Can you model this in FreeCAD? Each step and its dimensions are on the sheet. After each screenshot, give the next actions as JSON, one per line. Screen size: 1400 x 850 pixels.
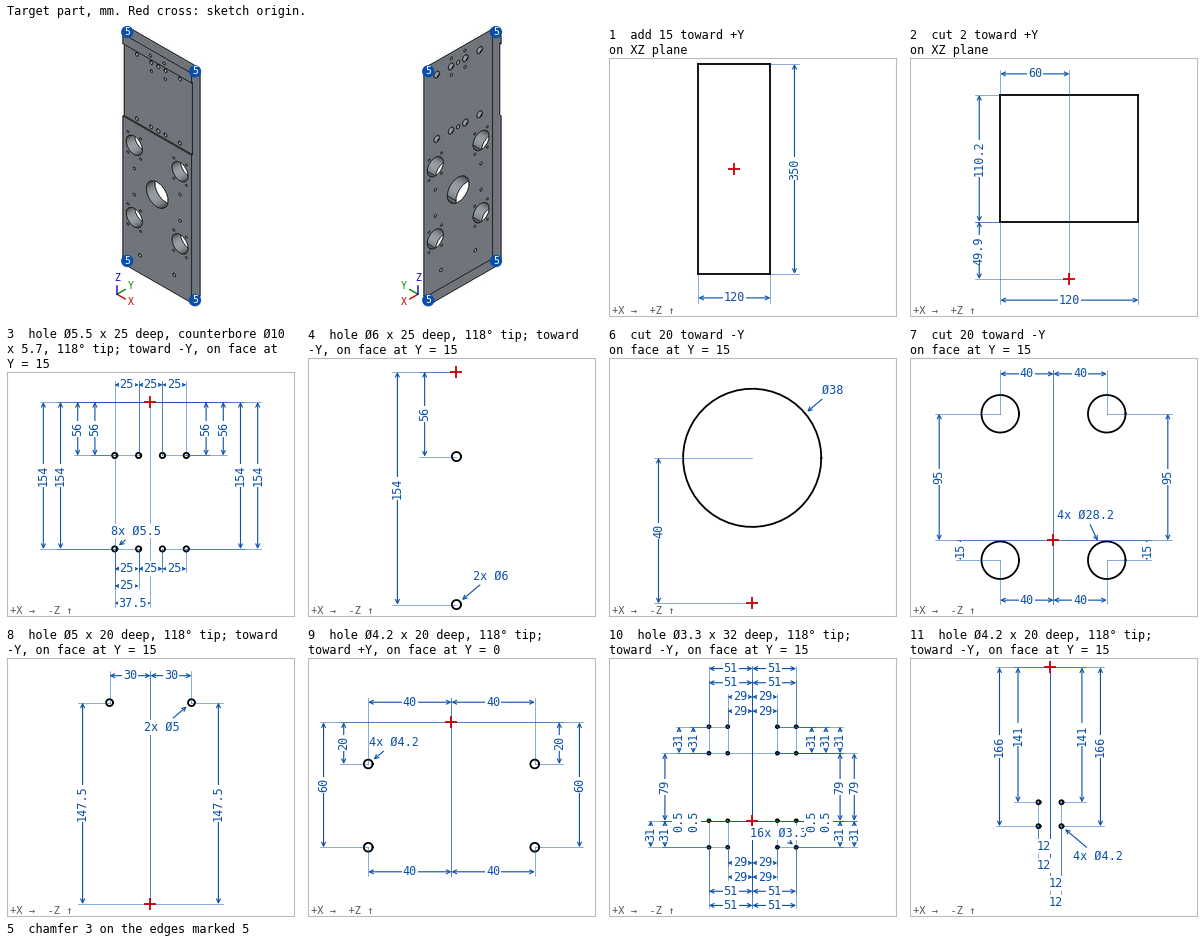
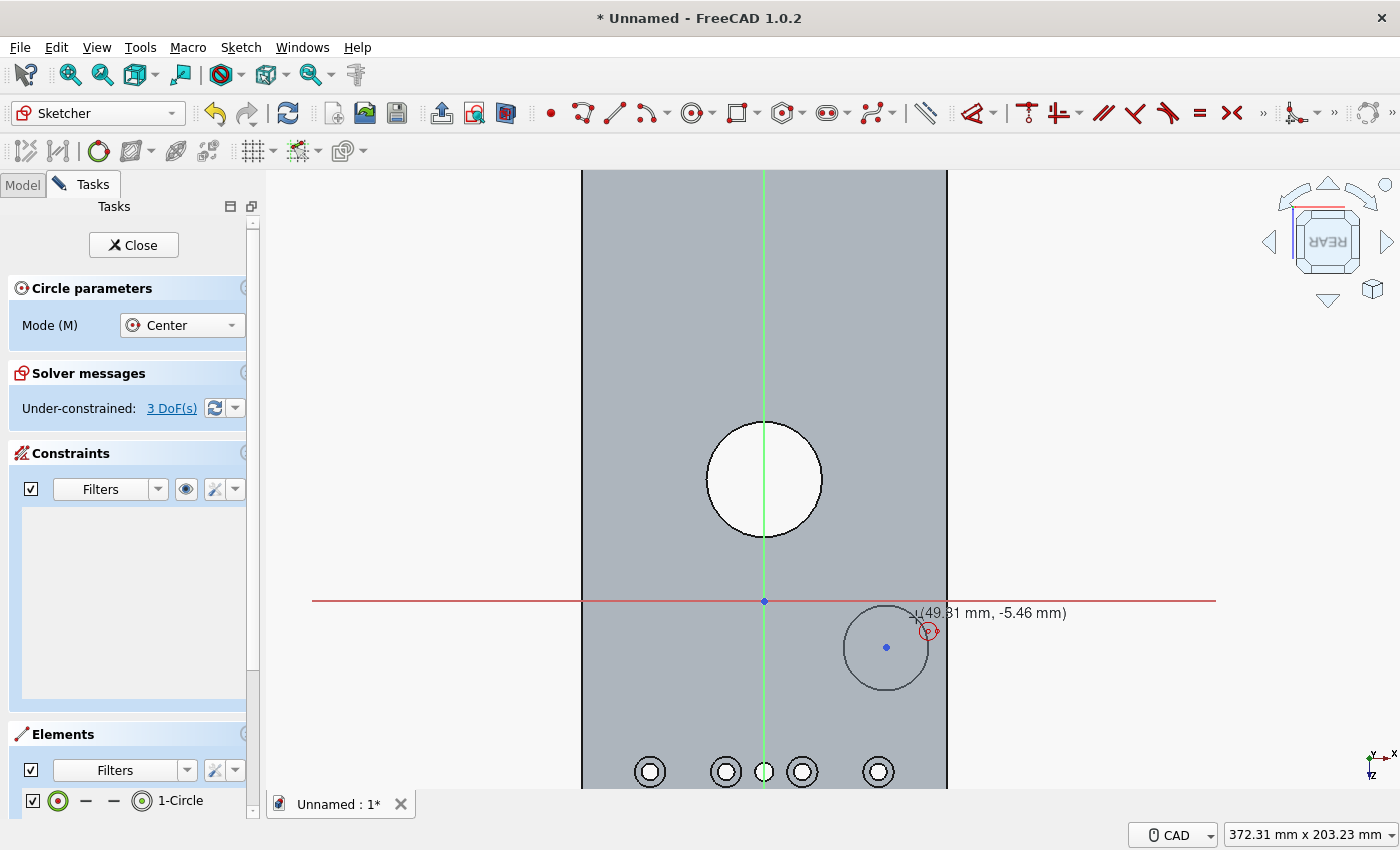
{"action": "left_click", "coordinate": [886, 312]}
{"action": "left_click", "coordinate": [916, 282]}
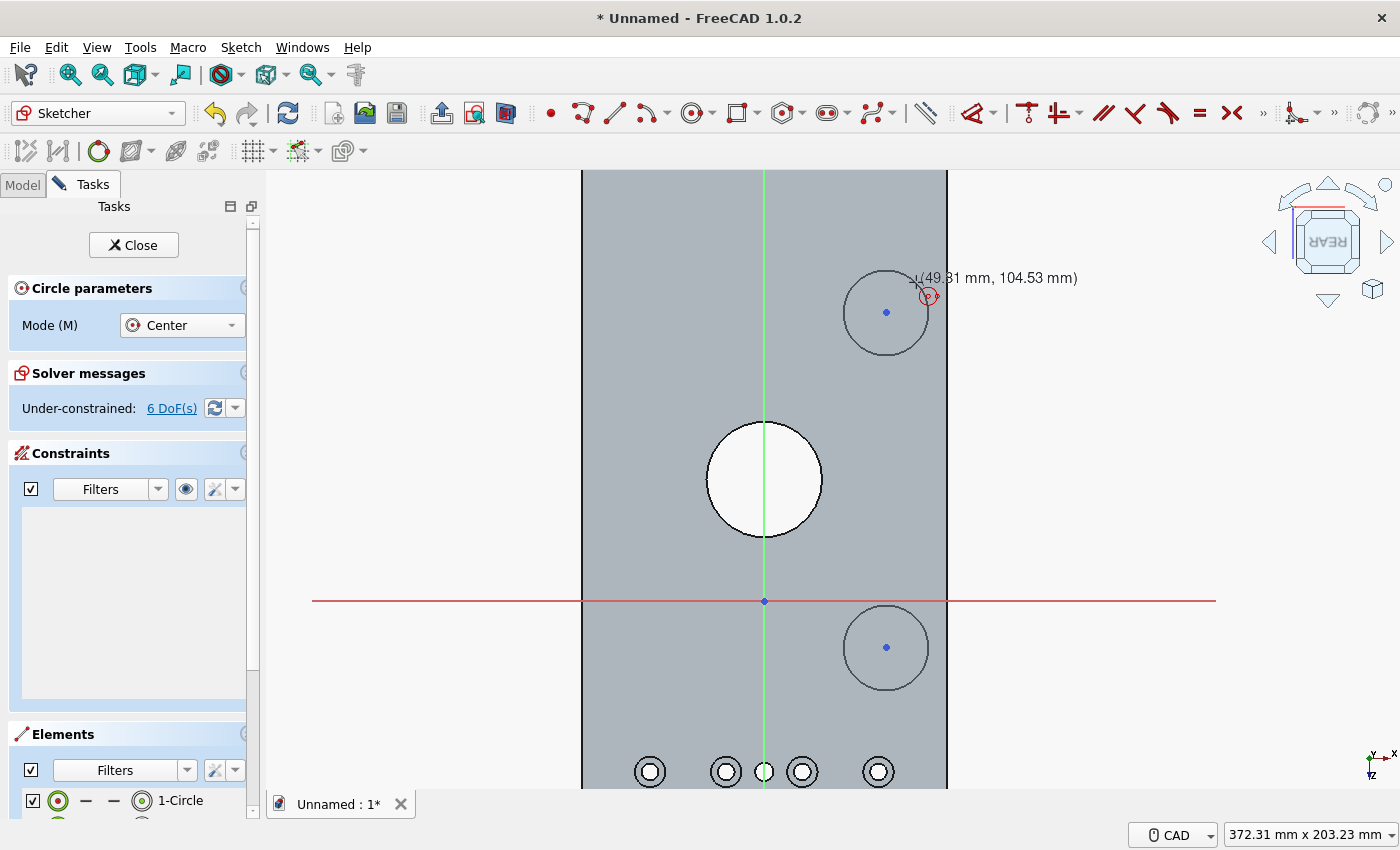
{"action": "left_click", "coordinate": [642, 647]}
{"action": "left_click", "coordinate": [673, 617]}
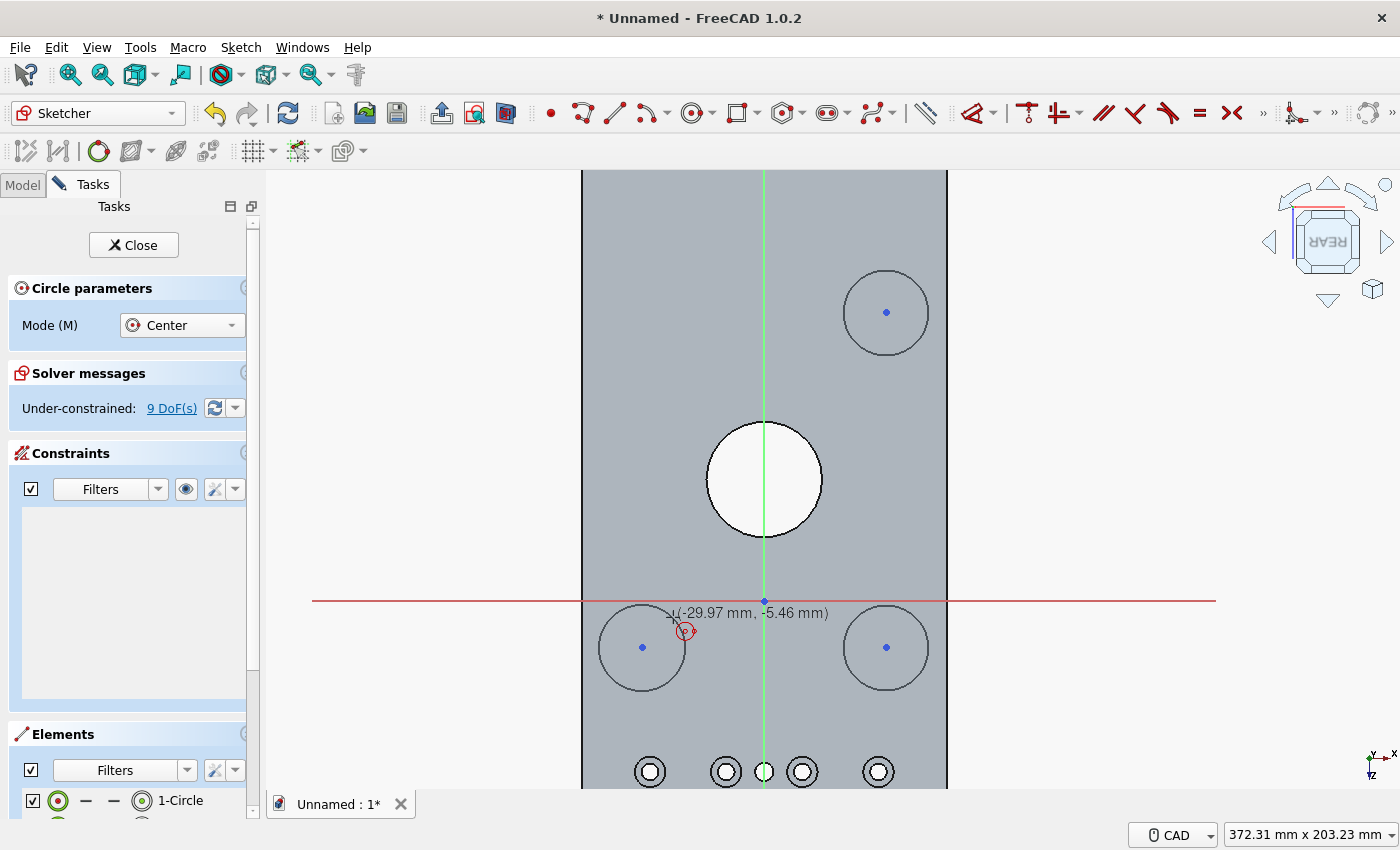
{"action": "left_click", "coordinate": [642, 312]}
{"action": "left_click", "coordinate": [673, 282]}
{"action": "key", "text": "Escape"}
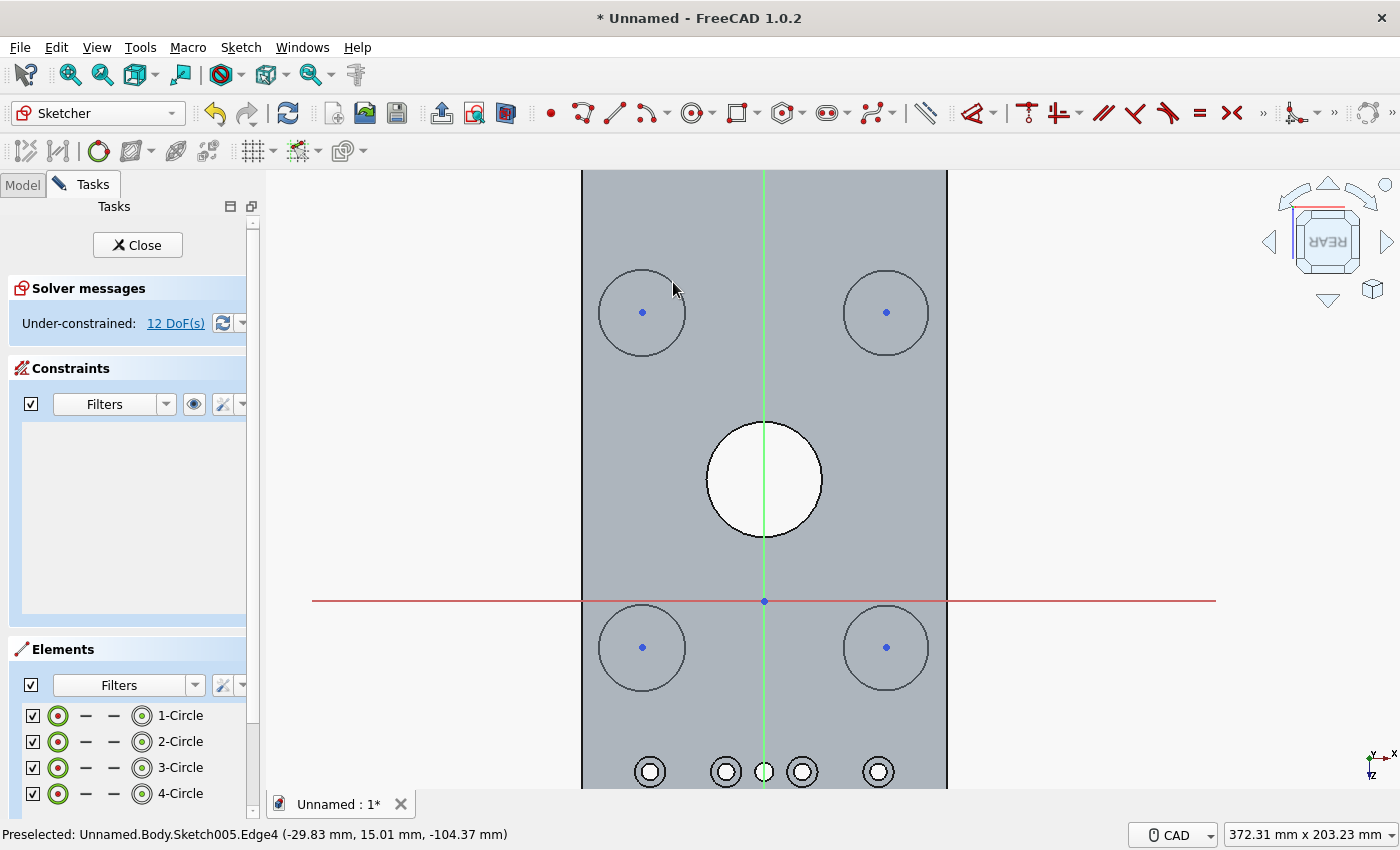
{"action": "left_click", "coordinate": [916, 618]}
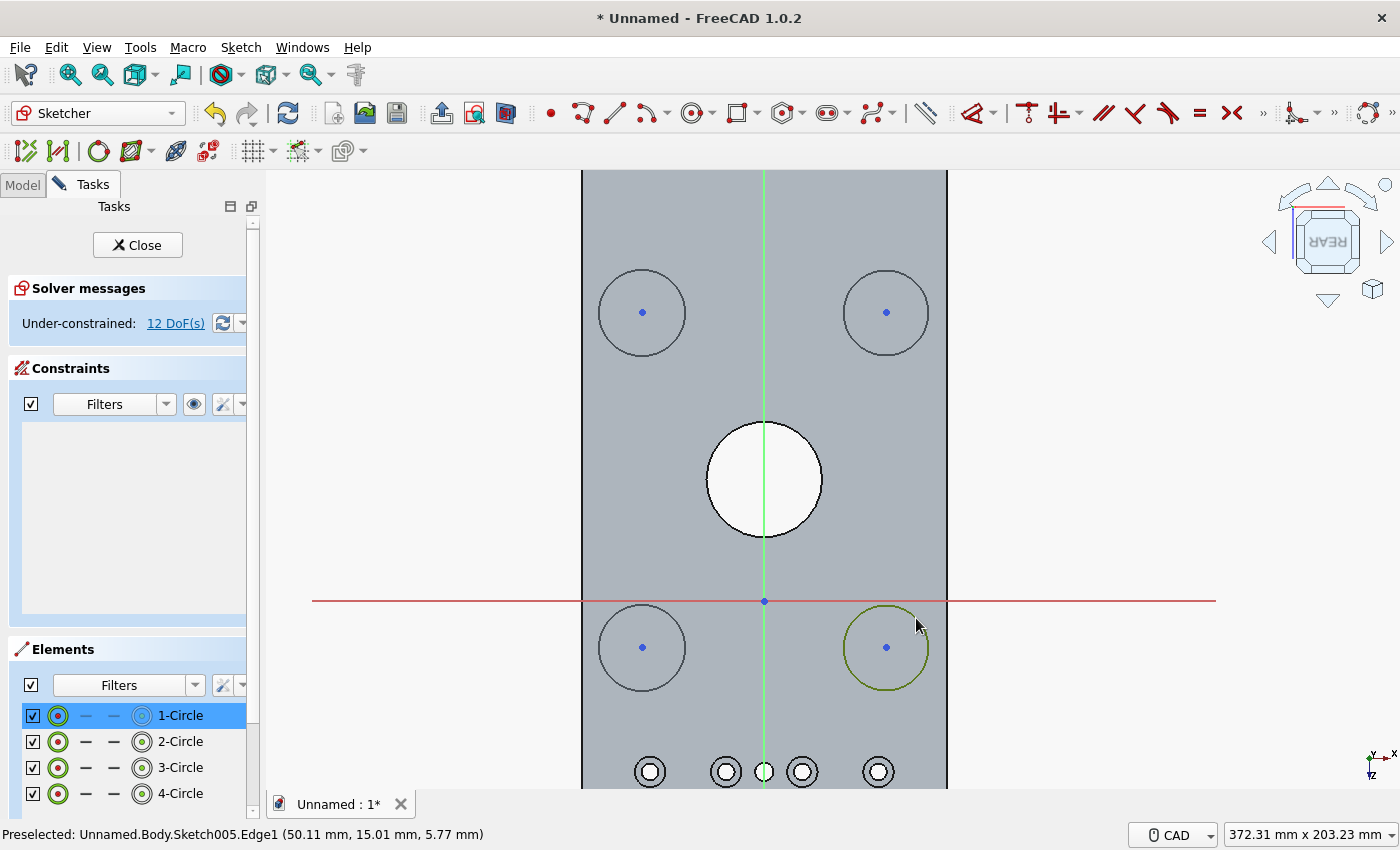
{"action": "left_click", "coordinate": [916, 283]}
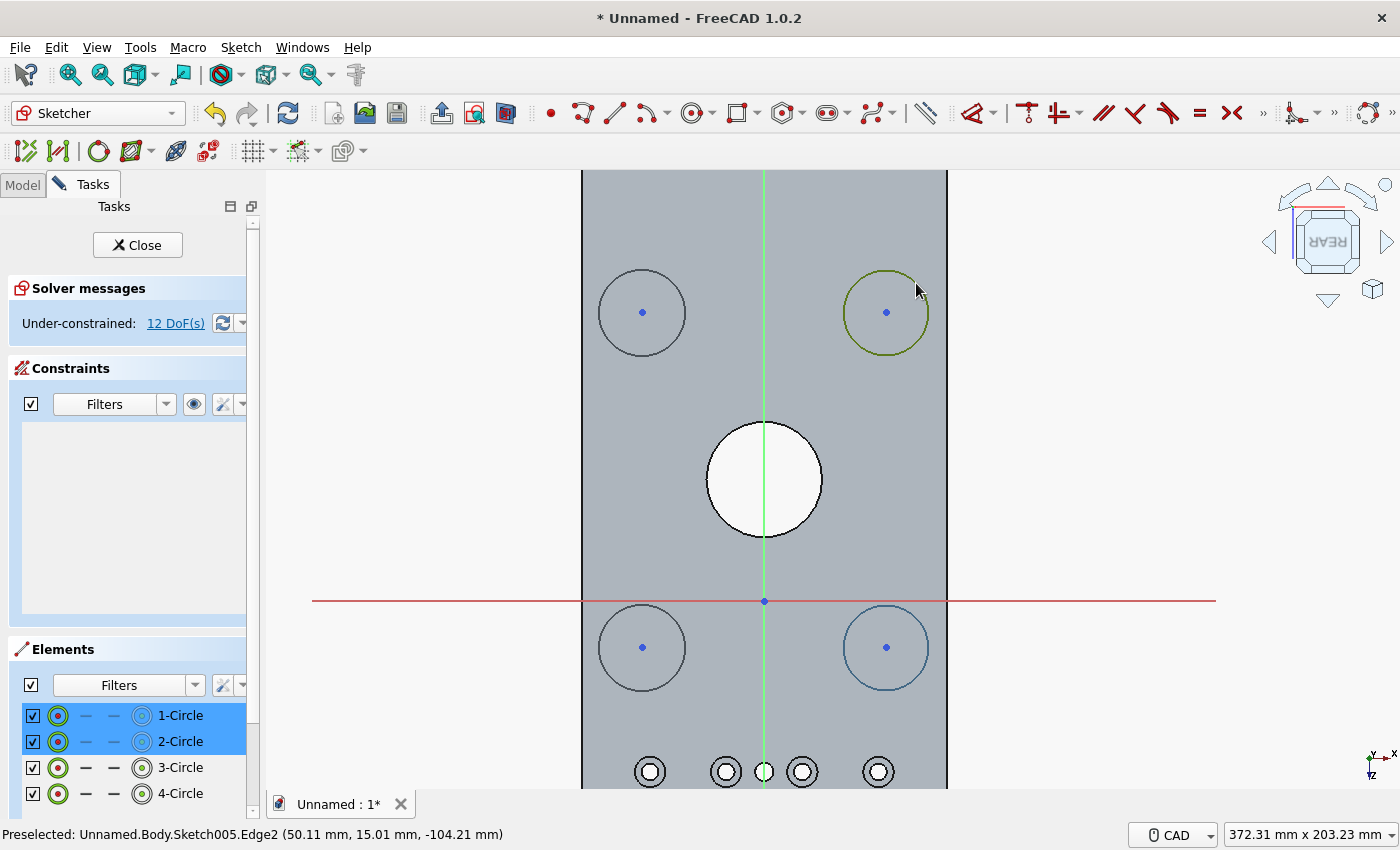
{"action": "left_click", "coordinate": [672, 617]}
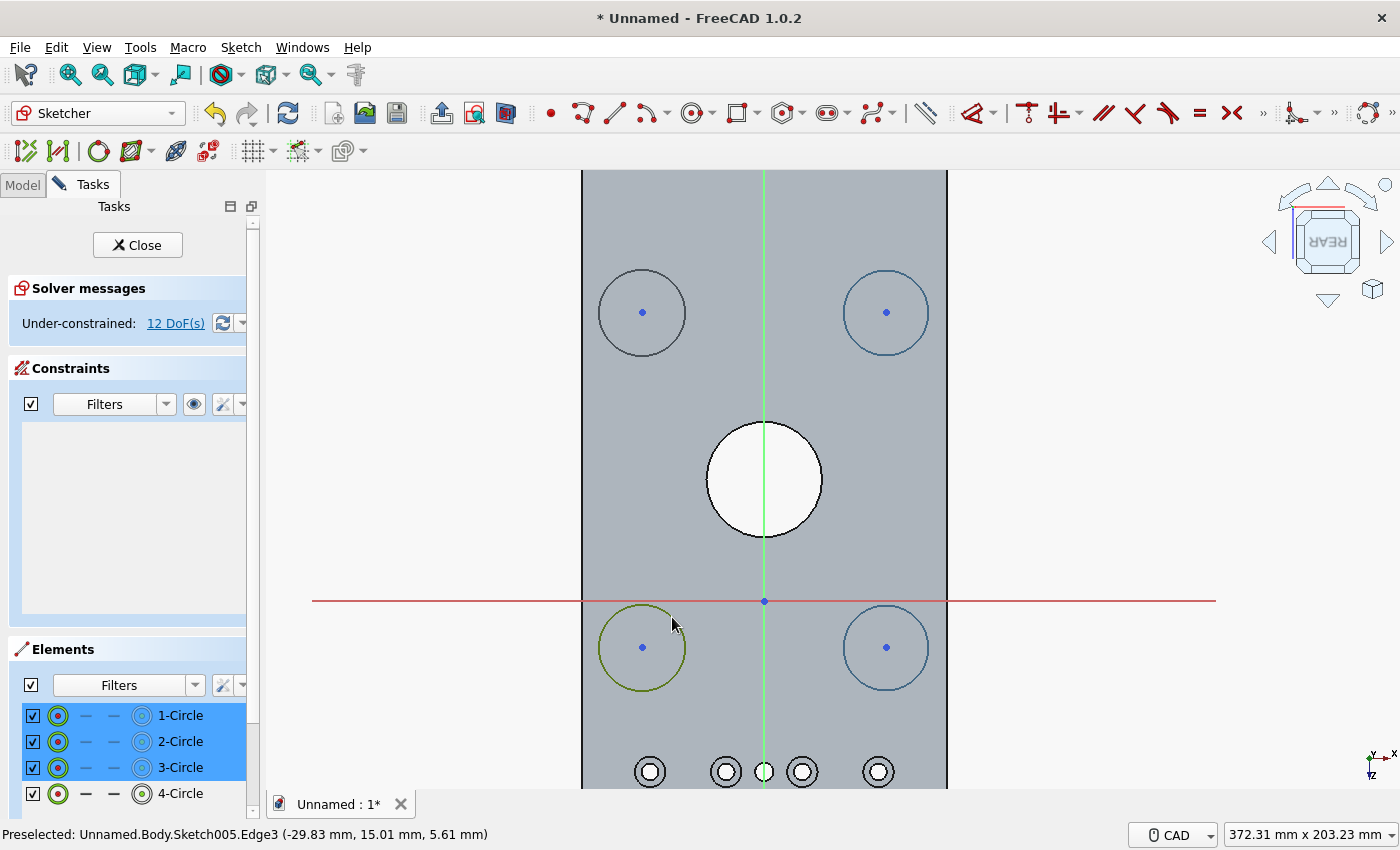
{"action": "left_click", "coordinate": [672, 282]}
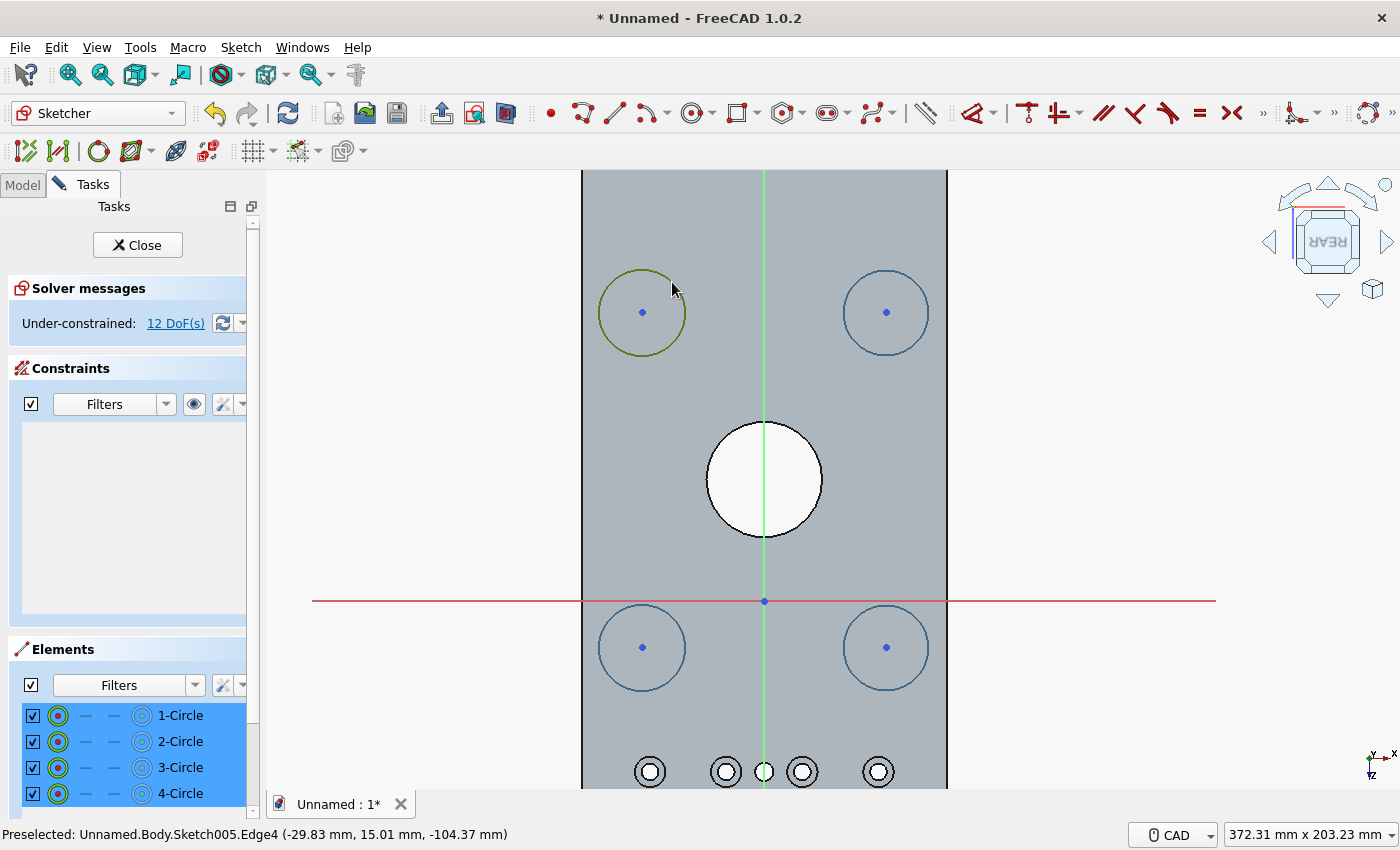
{"action": "left_click", "coordinate": [1200, 114]}